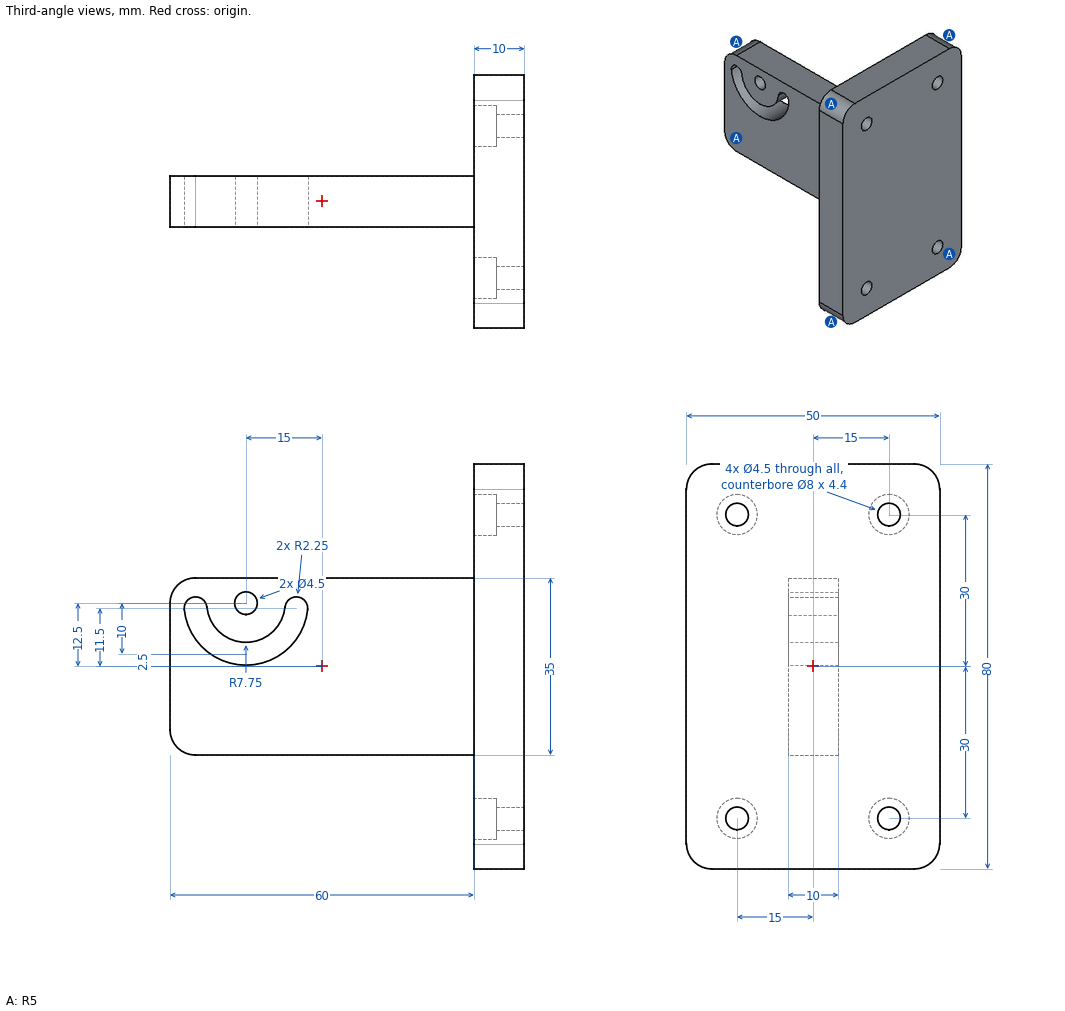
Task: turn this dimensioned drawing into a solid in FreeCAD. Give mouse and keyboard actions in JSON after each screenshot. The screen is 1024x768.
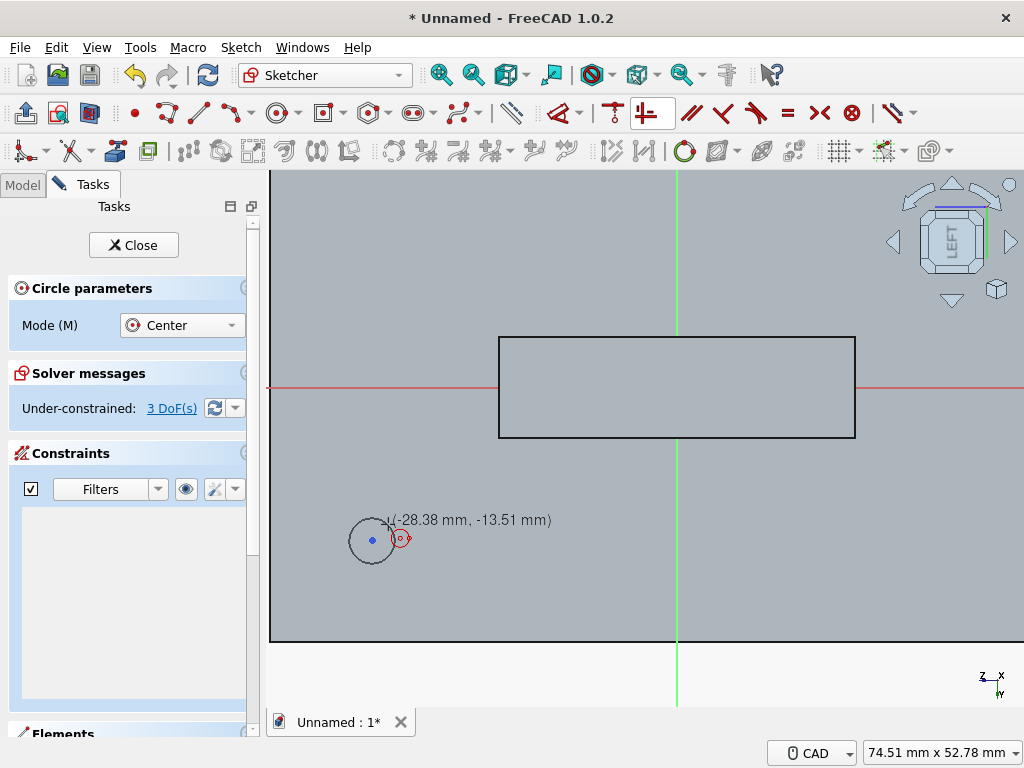
{"action": "scroll", "coordinate": [373, 542], "scroll_direction": "down", "scroll_amount": 2}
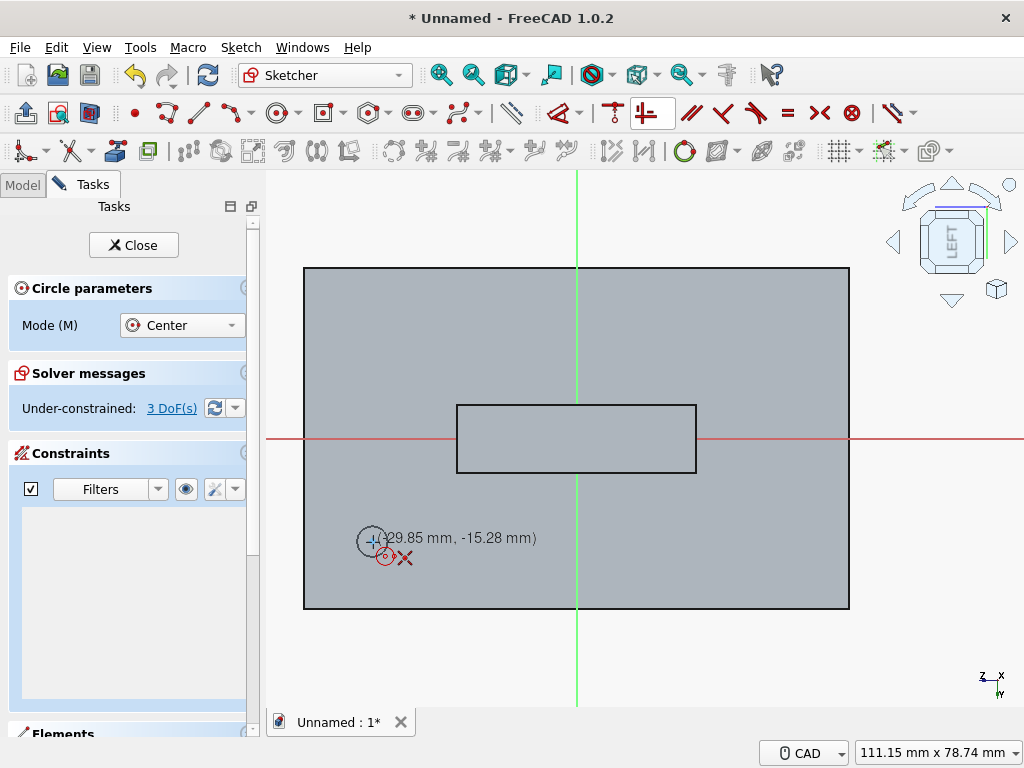
{"action": "scroll", "coordinate": [781, 541], "scroll_direction": "up", "scroll_amount": 2}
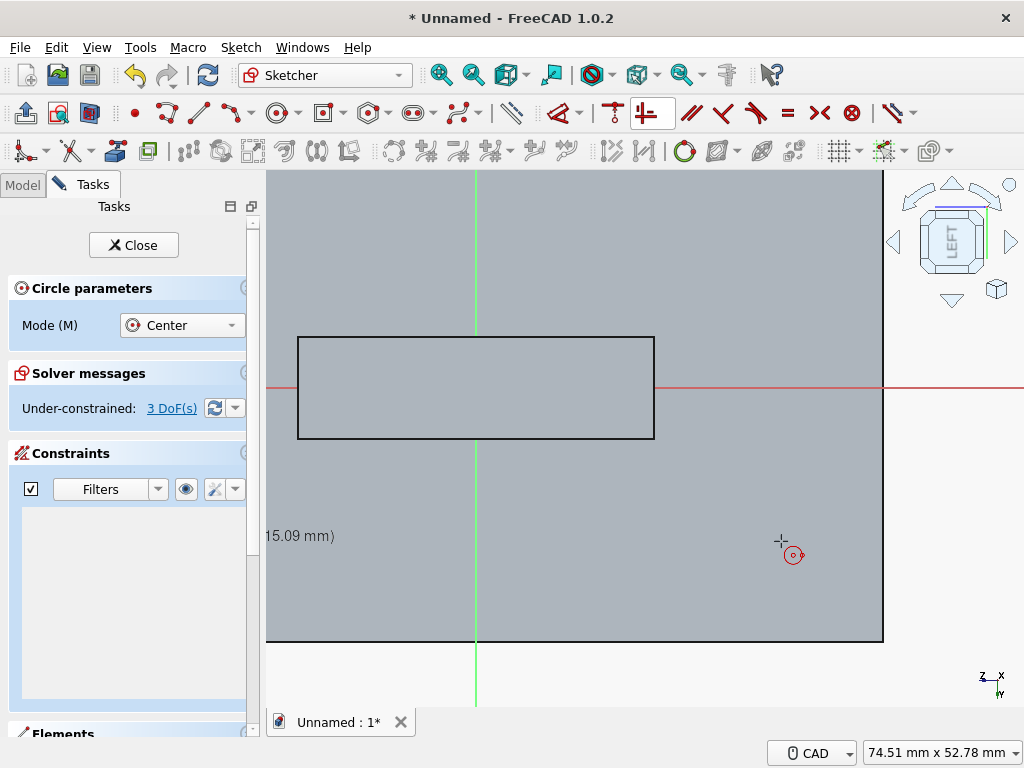
{"action": "left_click", "coordinate": [781, 541]}
{"action": "left_click", "coordinate": [797, 524]}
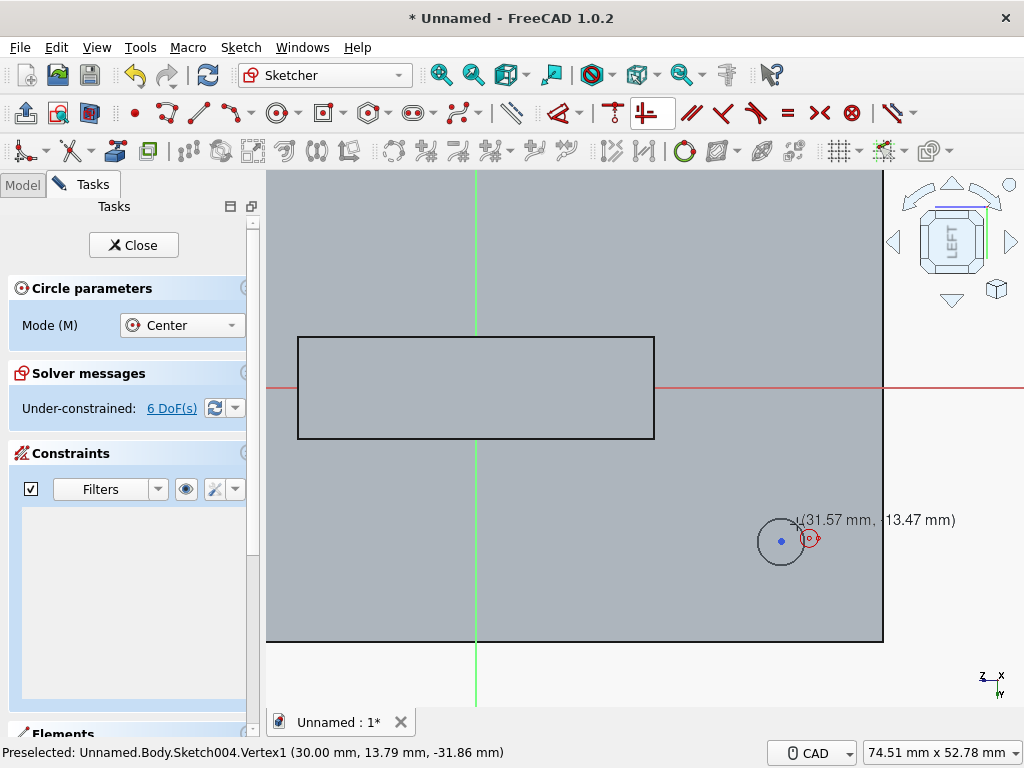
{"action": "left_click", "coordinate": [781, 235]}
{"action": "left_click", "coordinate": [797, 219]}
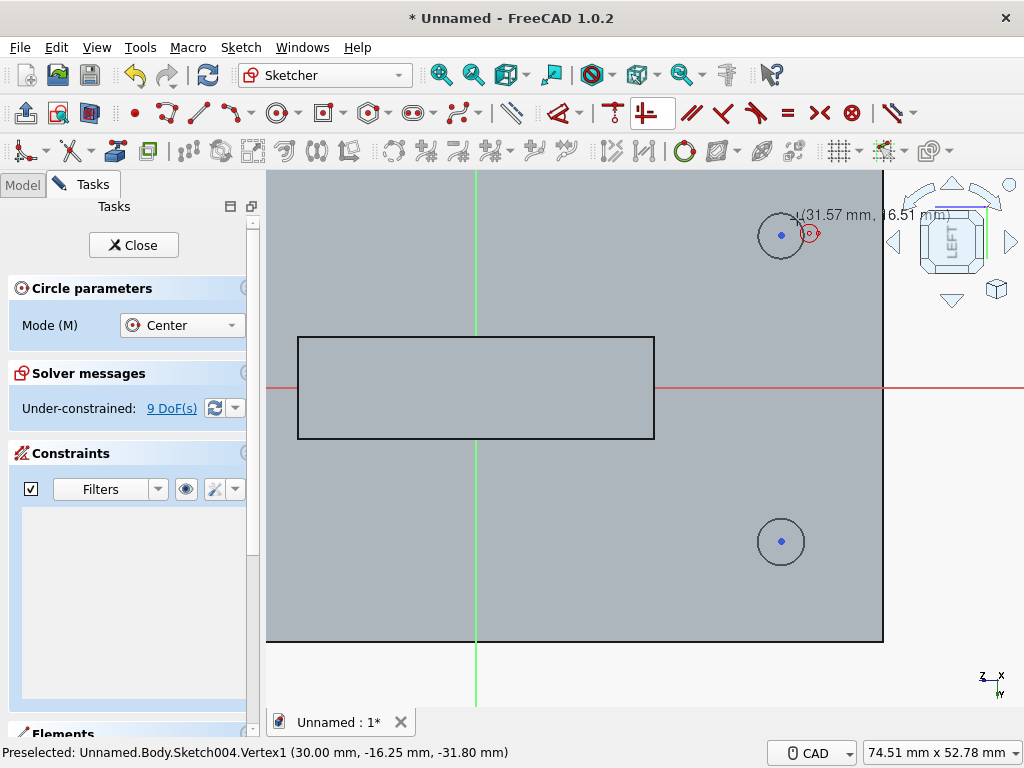
{"action": "scroll", "coordinate": [781, 541], "scroll_direction": "down", "scroll_amount": 2}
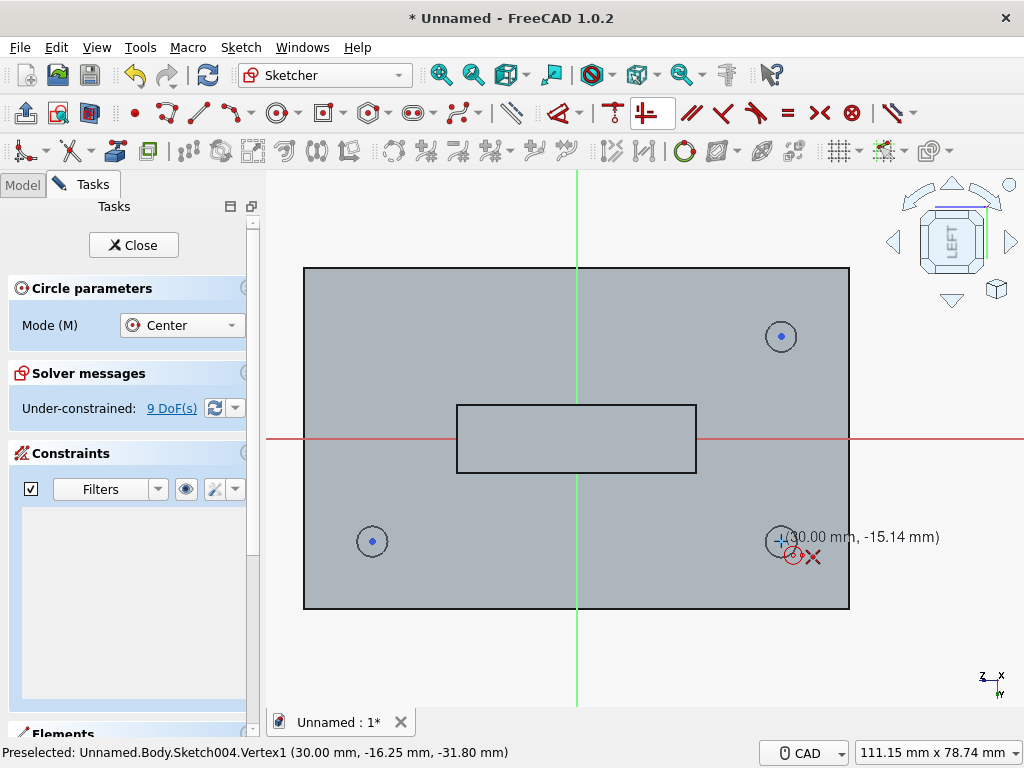
{"action": "scroll", "coordinate": [372, 336], "scroll_direction": "up", "scroll_amount": 2}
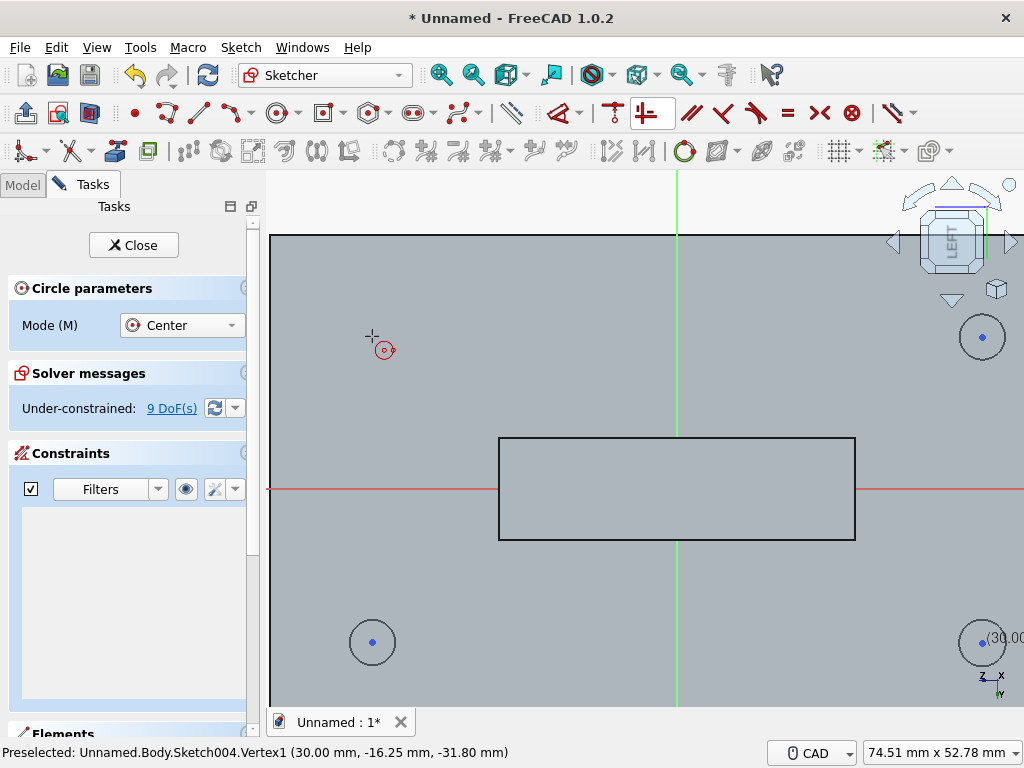
{"action": "left_click", "coordinate": [372, 336]}
{"action": "left_click", "coordinate": [388, 320]}
{"action": "key", "text": "Escape"}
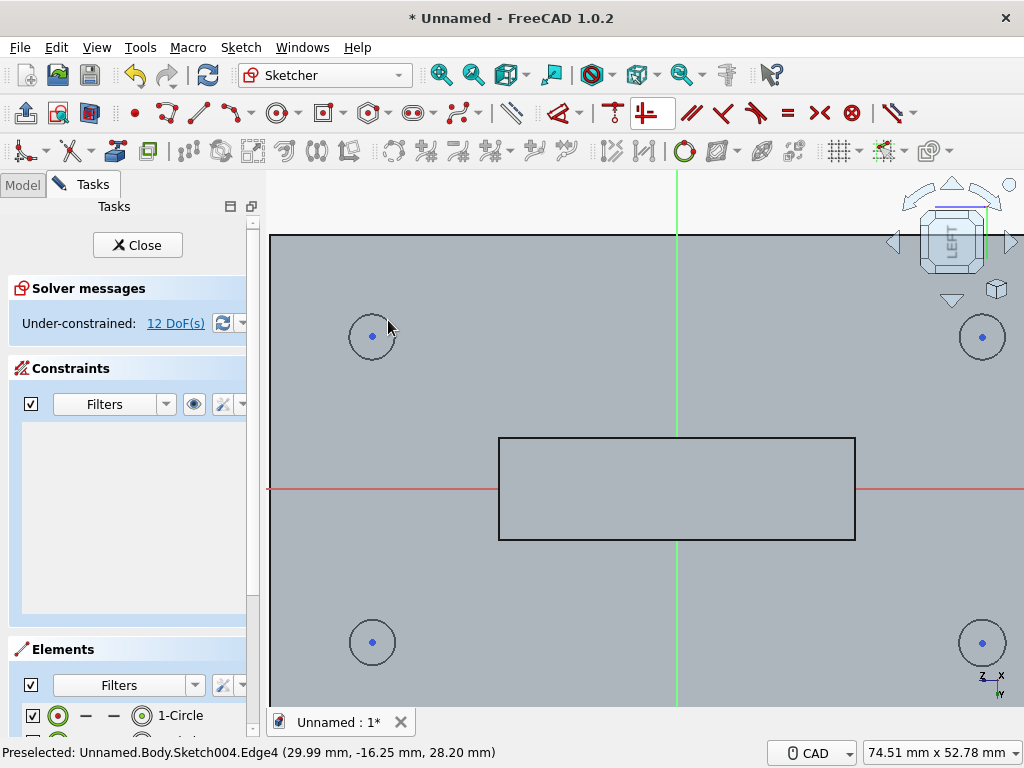
{"action": "left_click", "coordinate": [388, 626]}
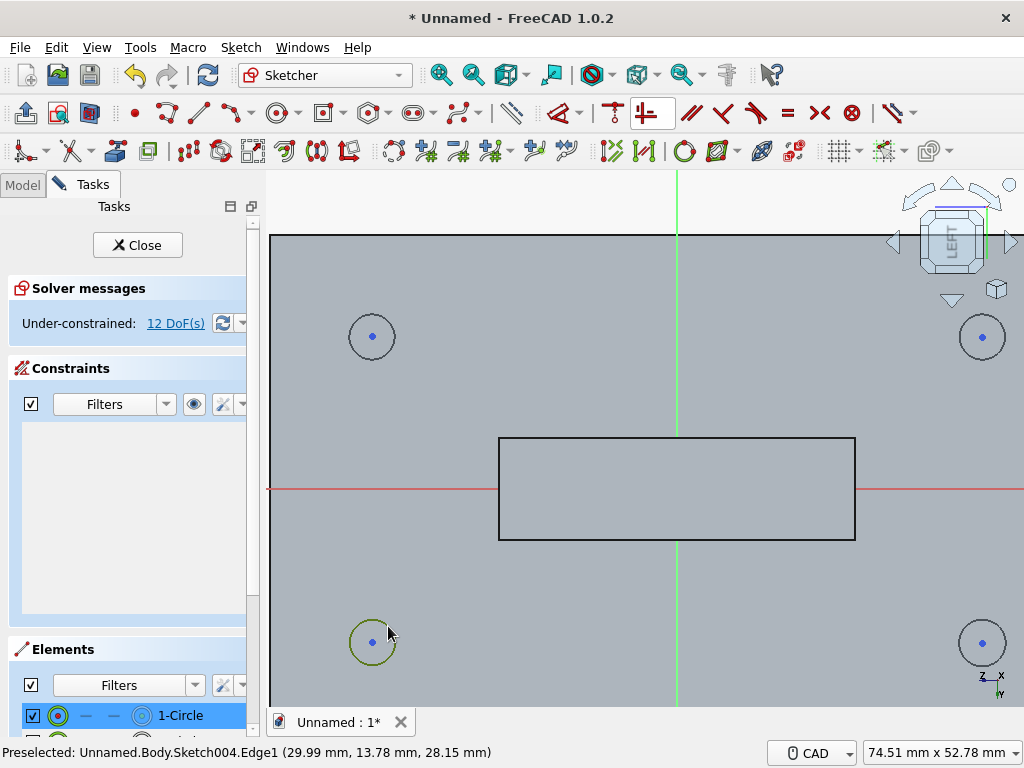
{"action": "scroll", "coordinate": [372, 336], "scroll_direction": "down", "scroll_amount": 2}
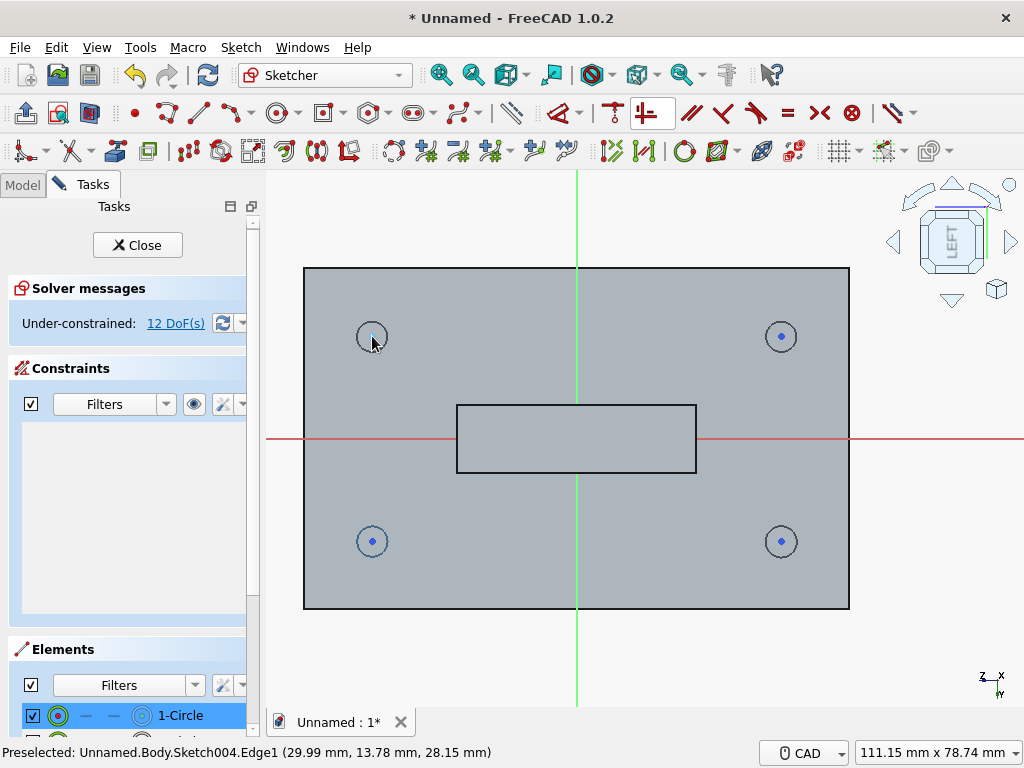
{"action": "left_click", "coordinate": [792, 531]}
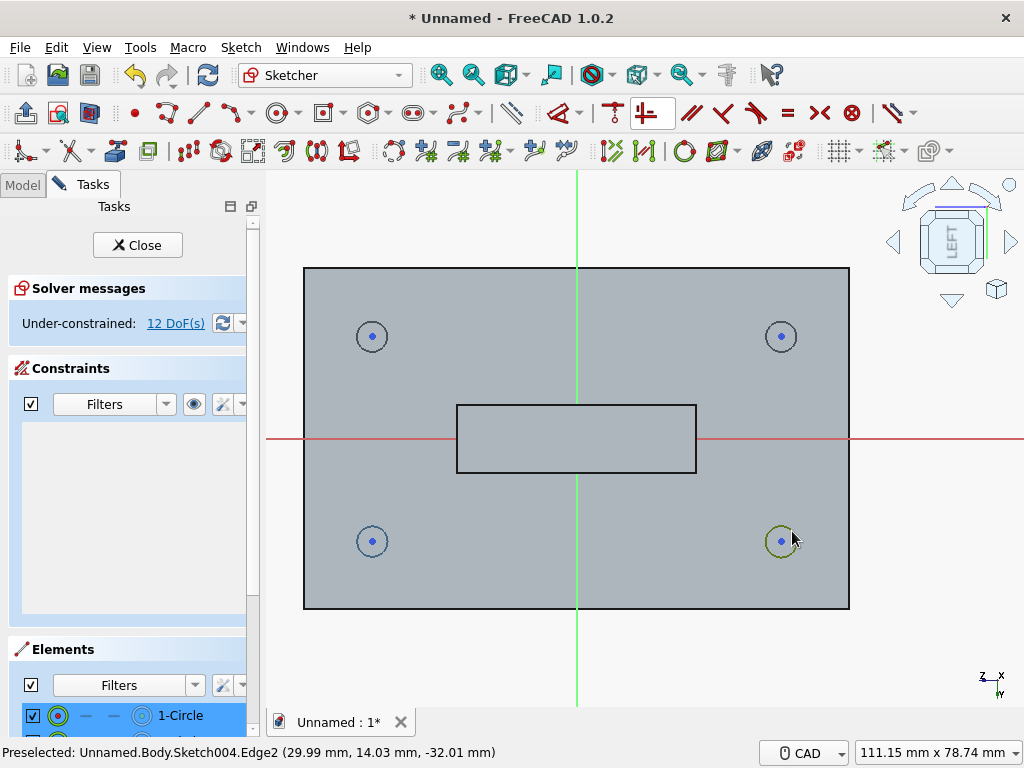
{"action": "left_click", "coordinate": [792, 326]}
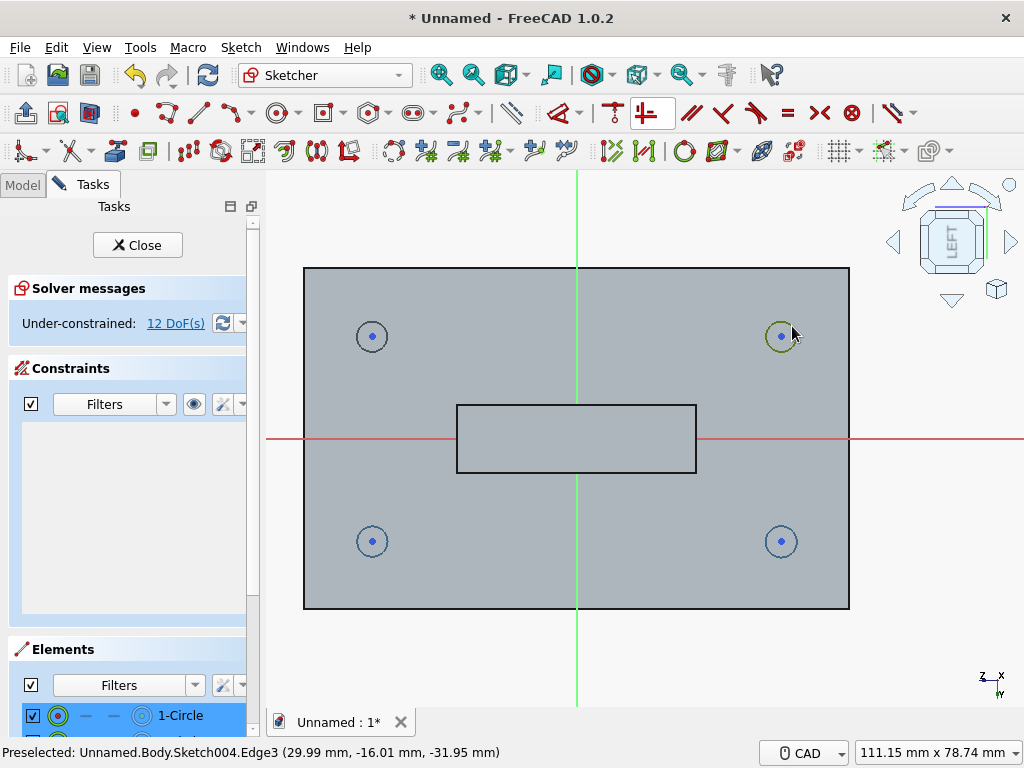
{"action": "left_click", "coordinate": [383, 326]}